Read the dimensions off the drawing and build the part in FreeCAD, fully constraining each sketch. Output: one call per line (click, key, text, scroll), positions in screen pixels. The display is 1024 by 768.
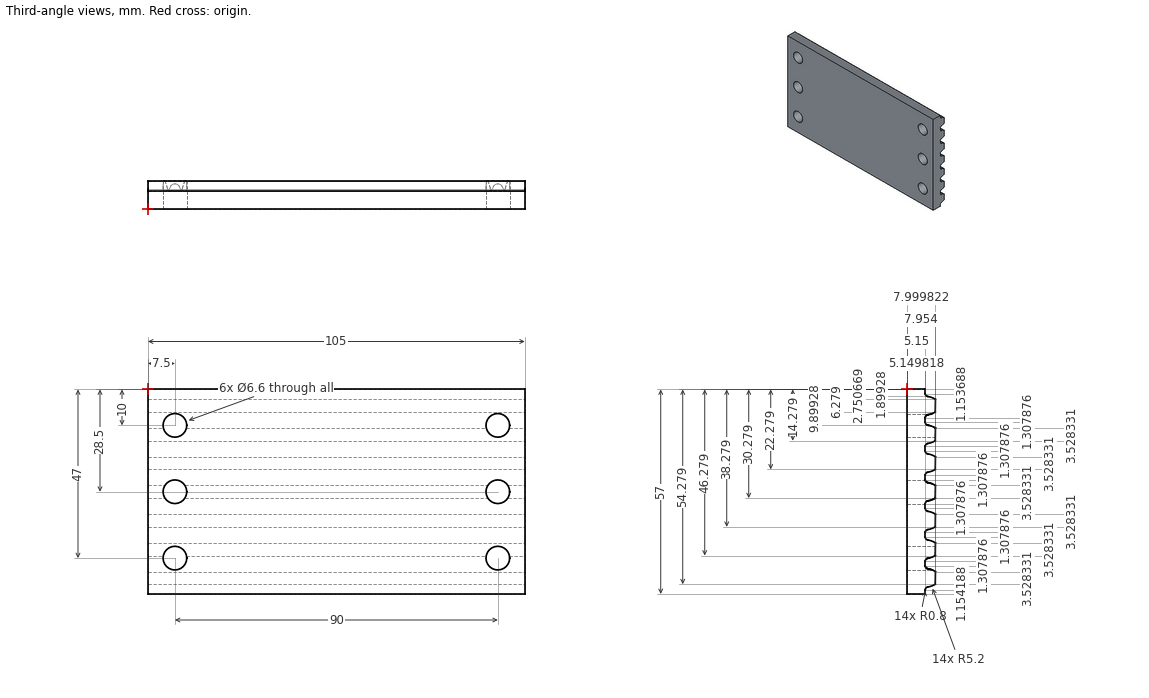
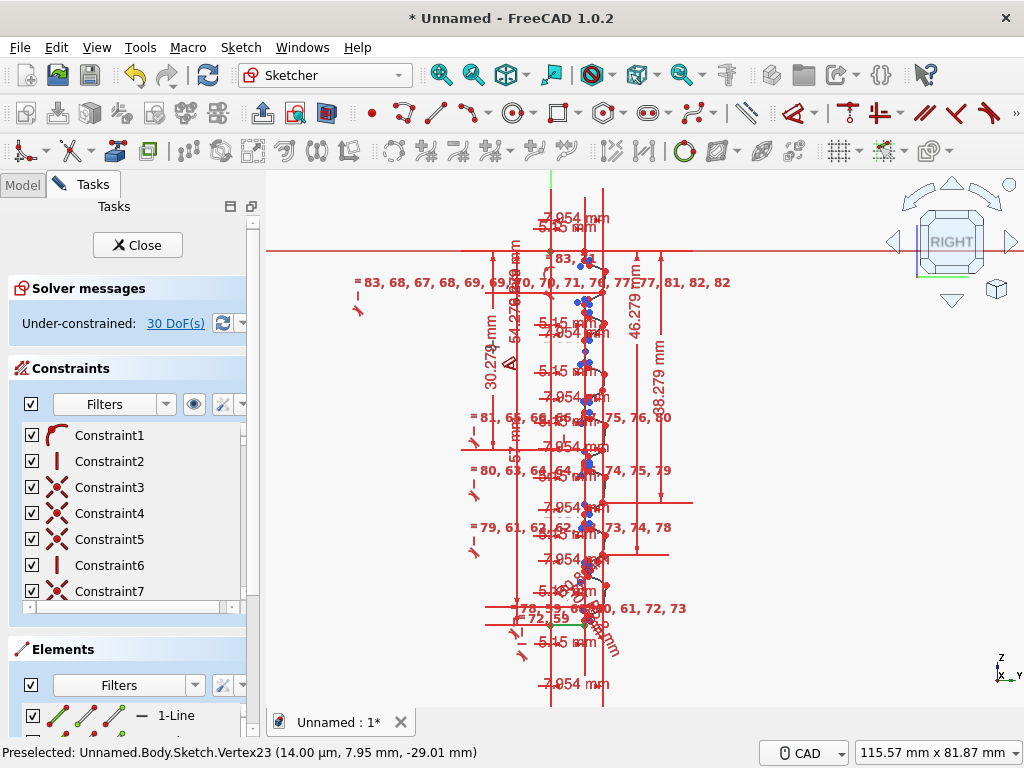
click(603, 390)
click(637, 272)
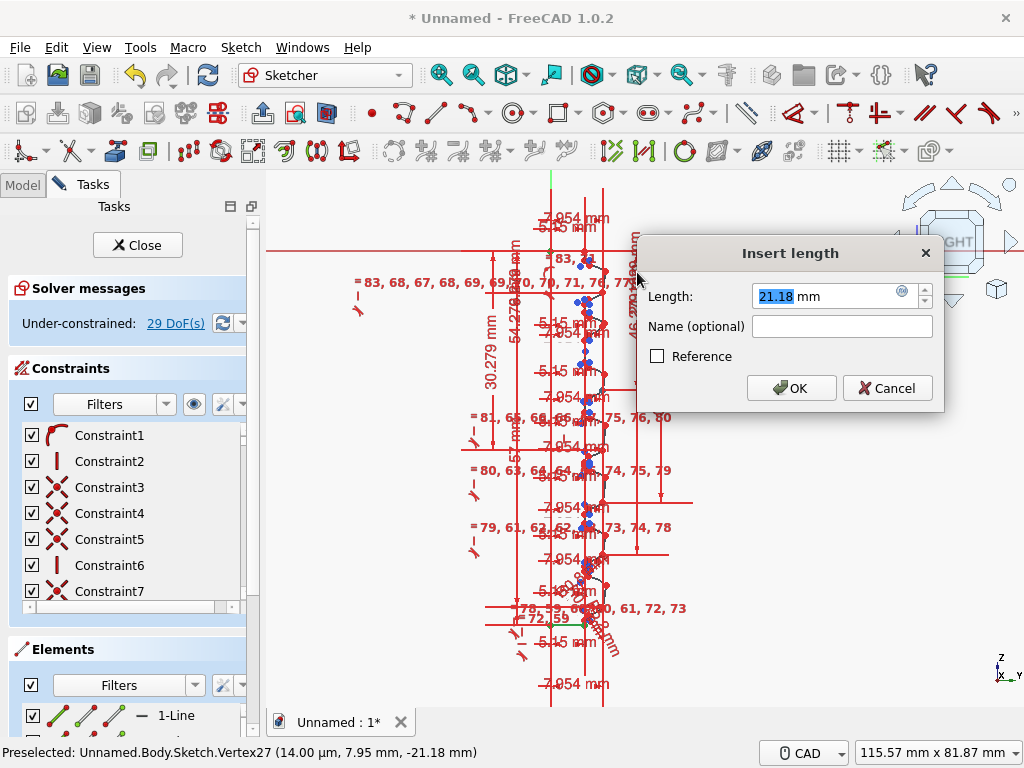
text(22.279)
key(Return)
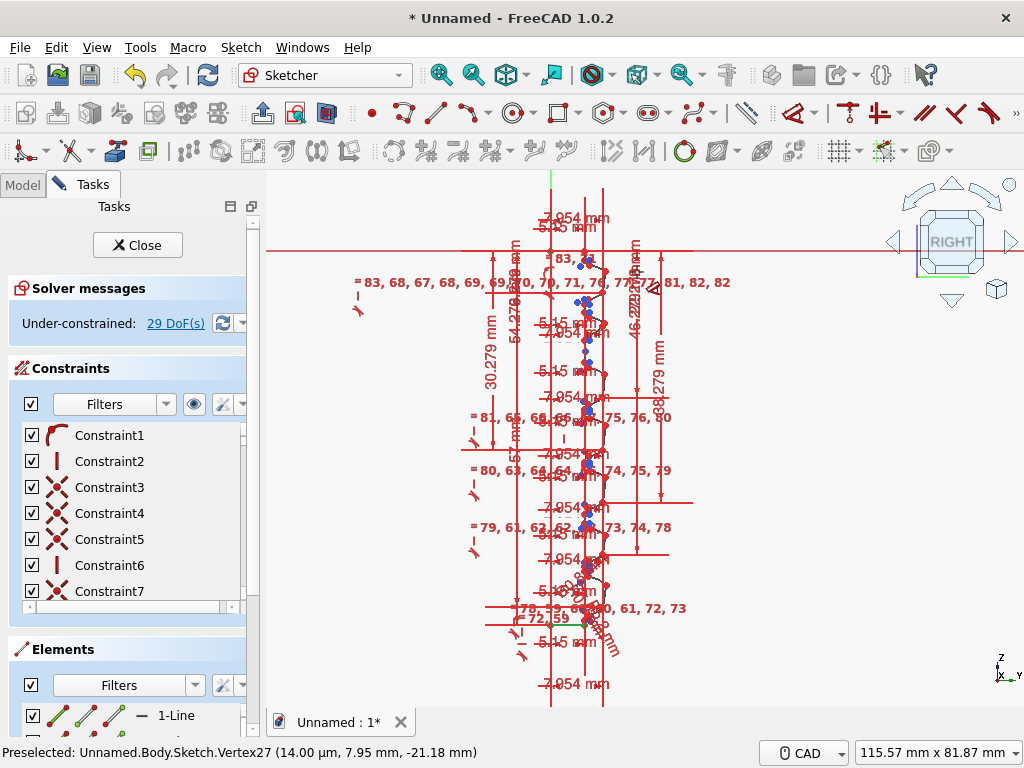
scroll(603, 326, up, 7)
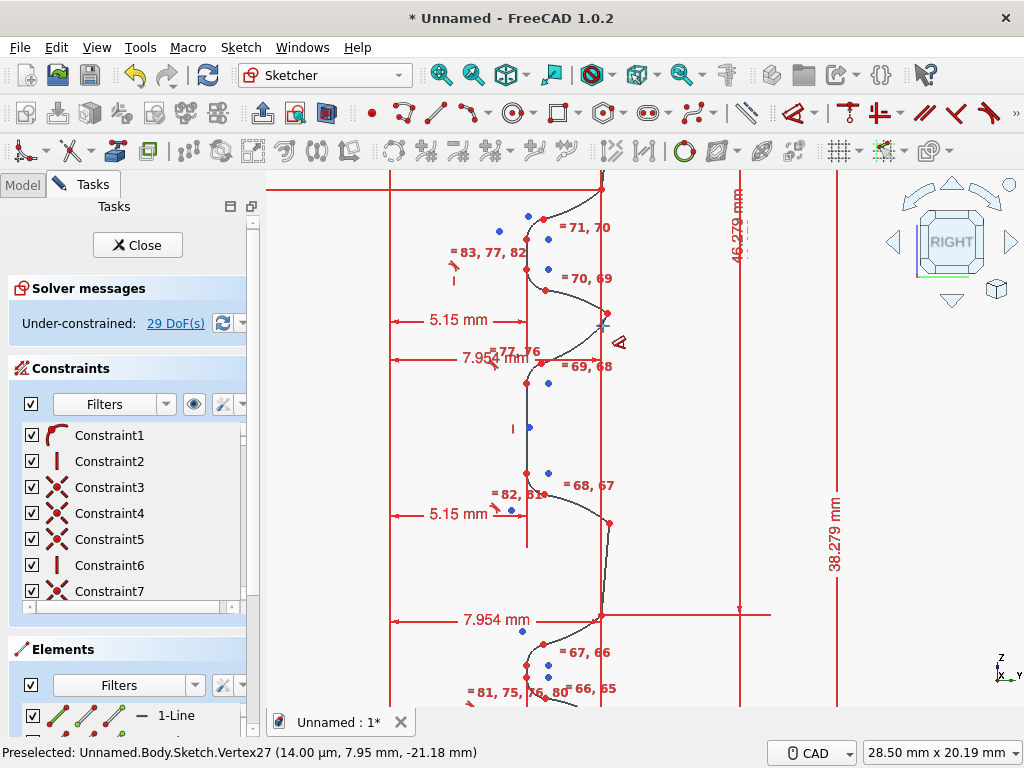
click(601, 325)
click(356, 262)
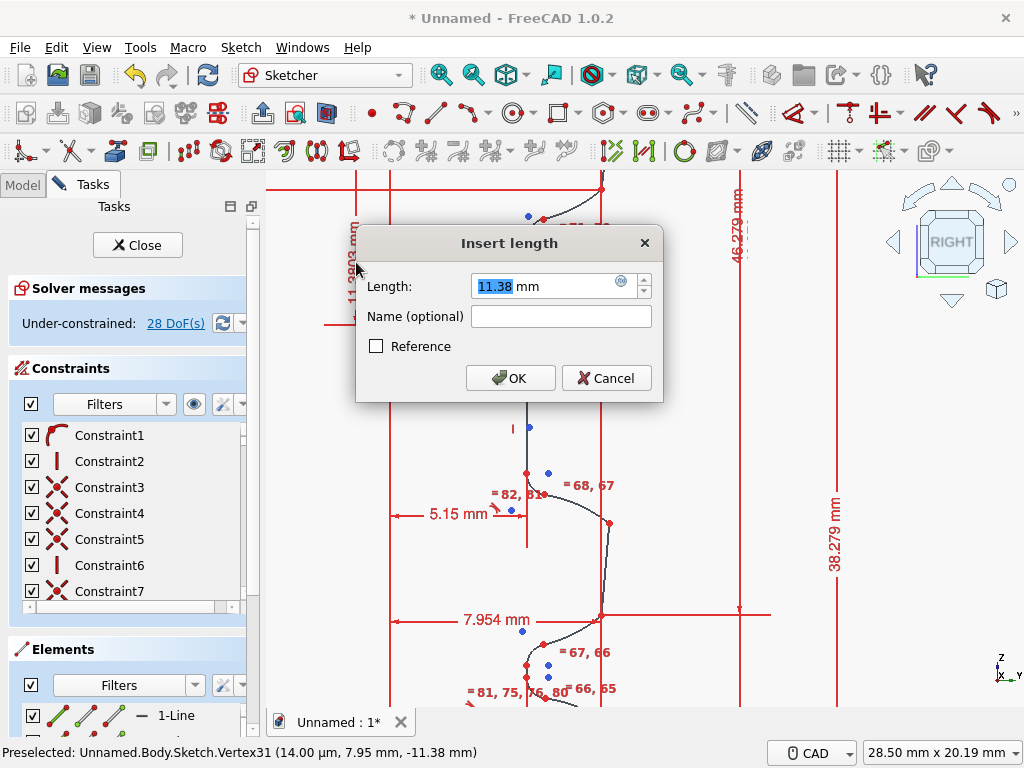
text(14.279)
key(Return)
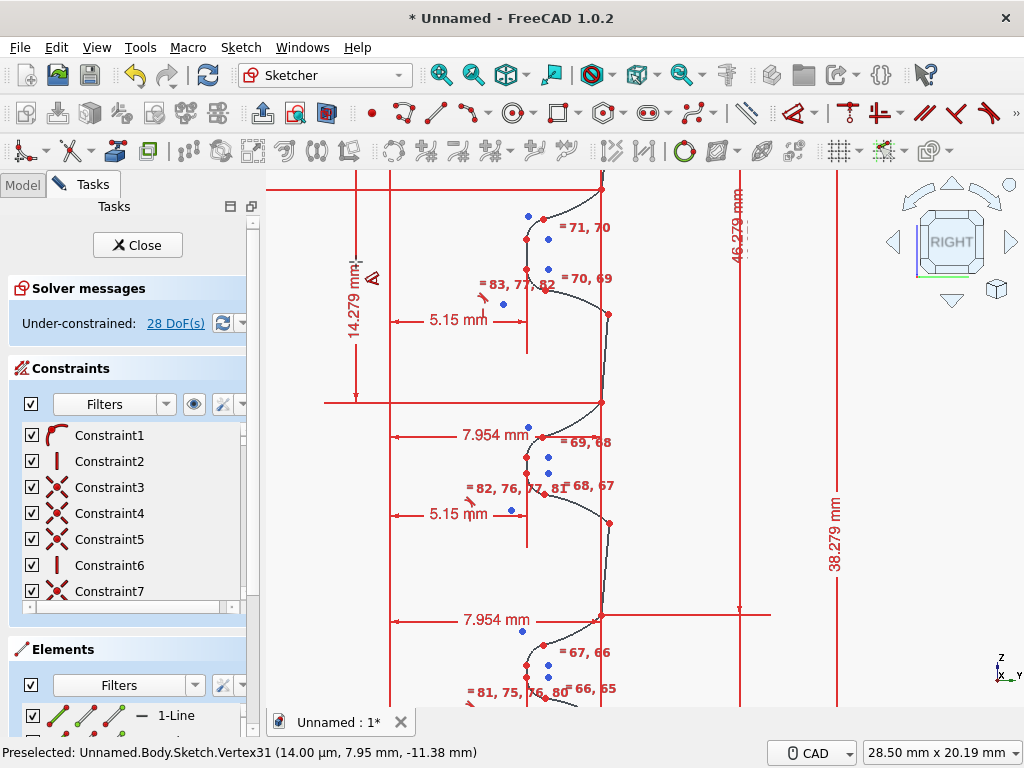
scroll(603, 326, down, 7)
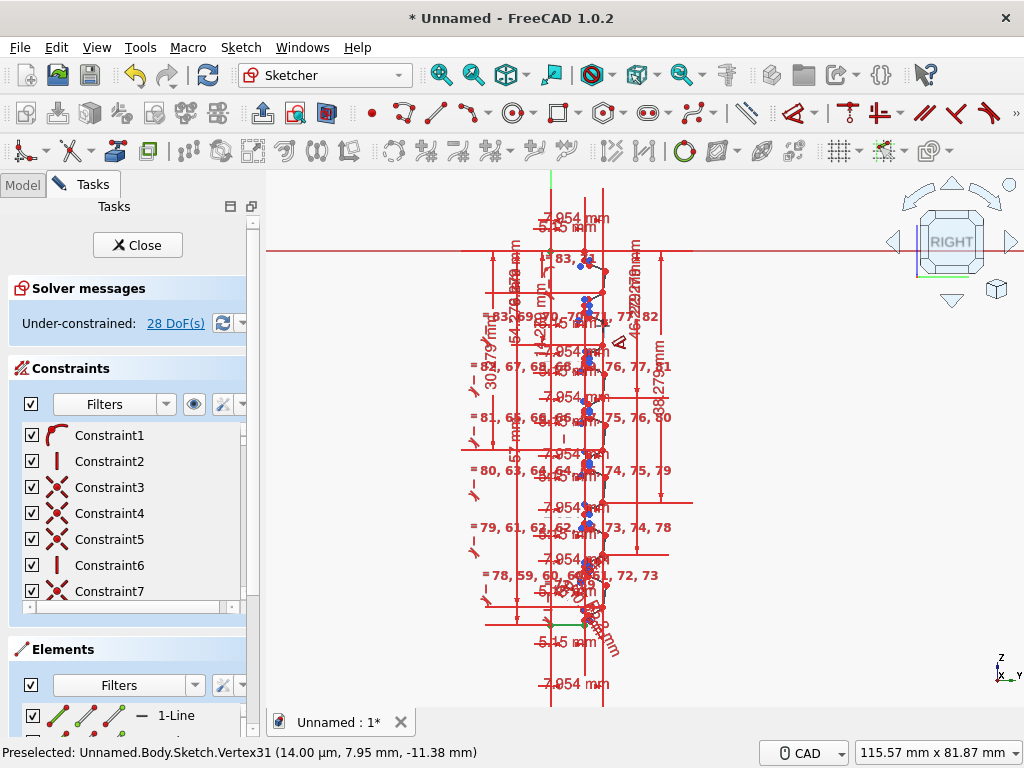
scroll(585, 257, up, 9)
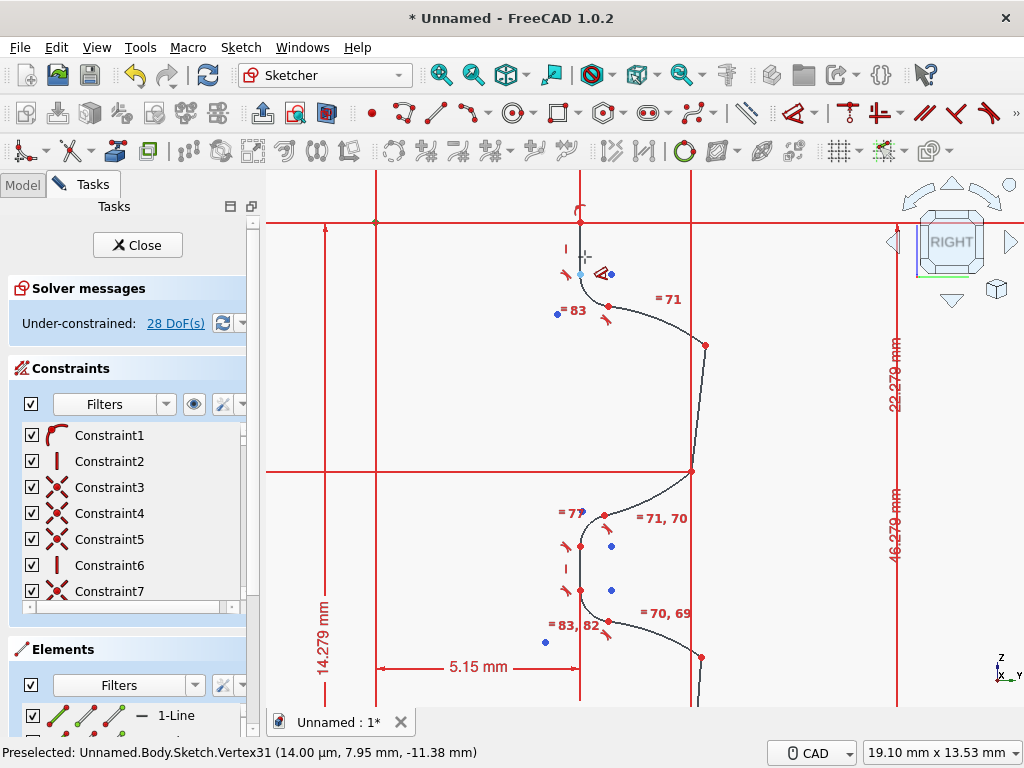
click(580, 259)
click(614, 249)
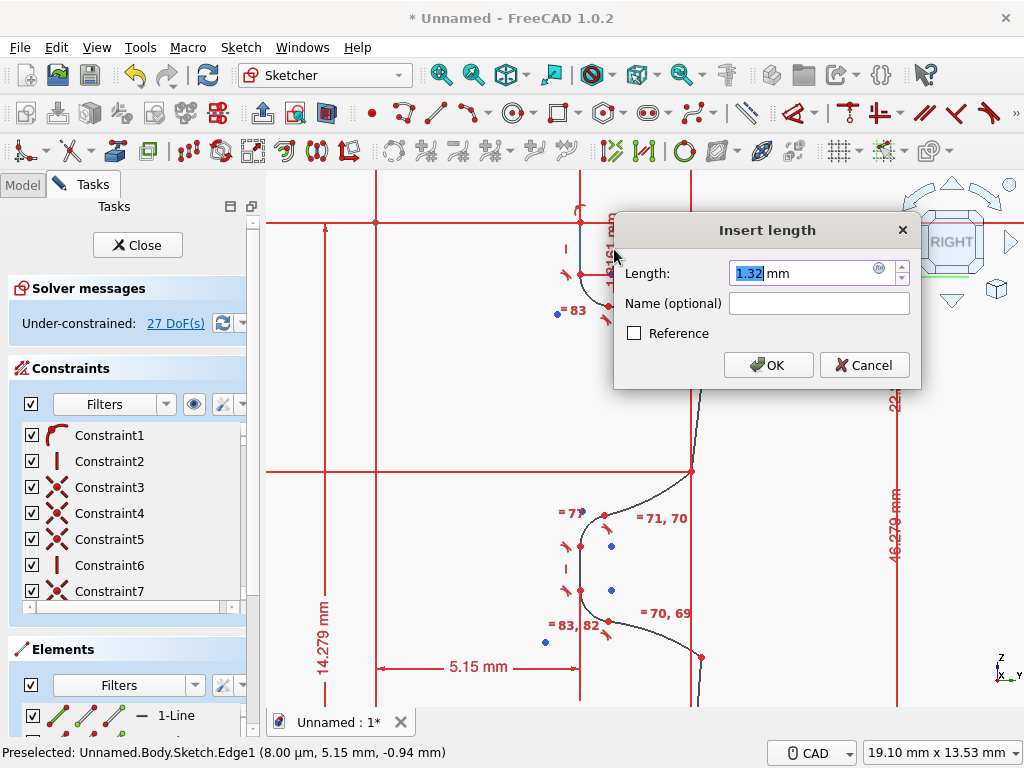
text(1.153688)
key(Return)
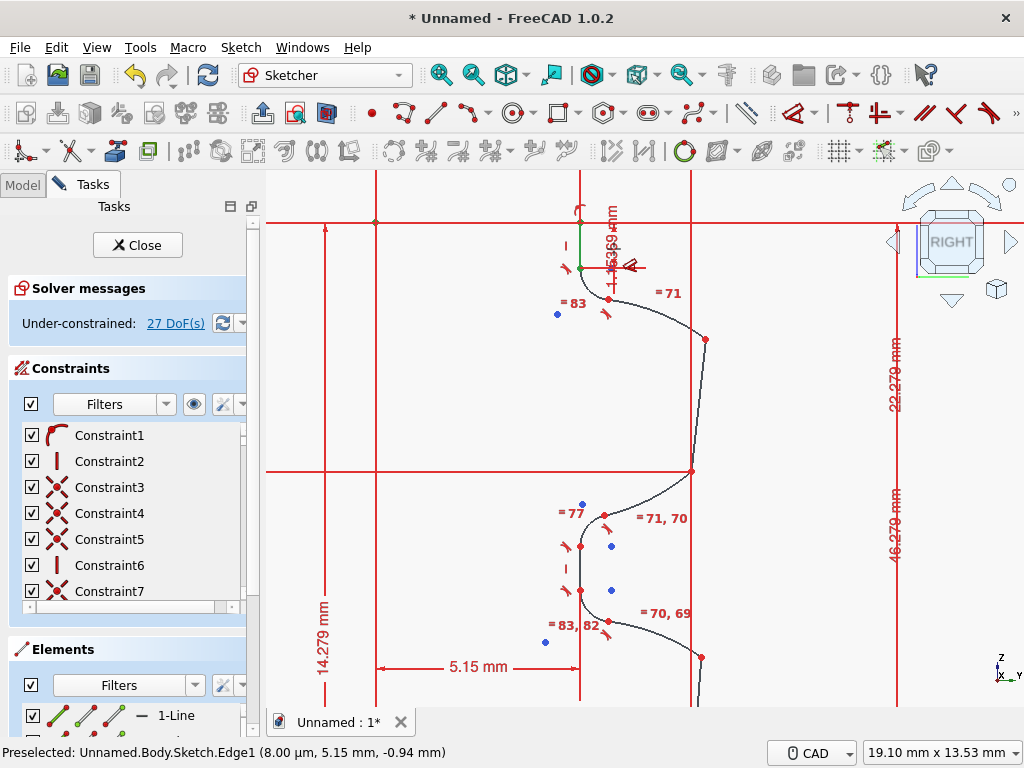
scroll(585, 257, down, 9)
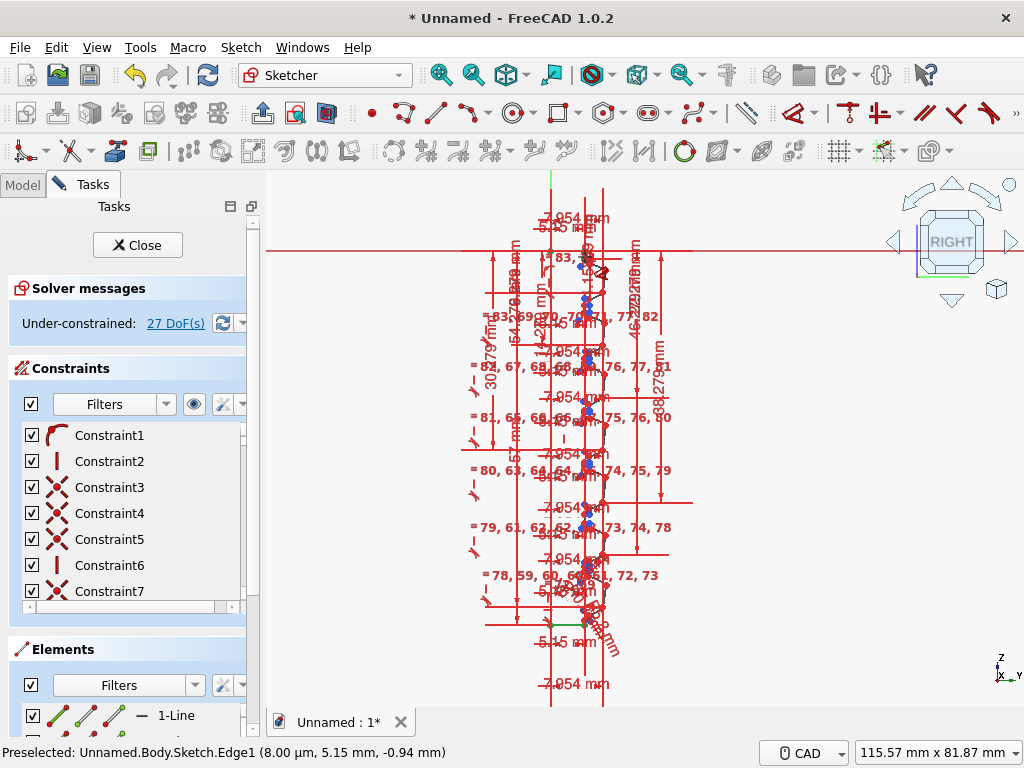
scroll(585, 624, up, 12)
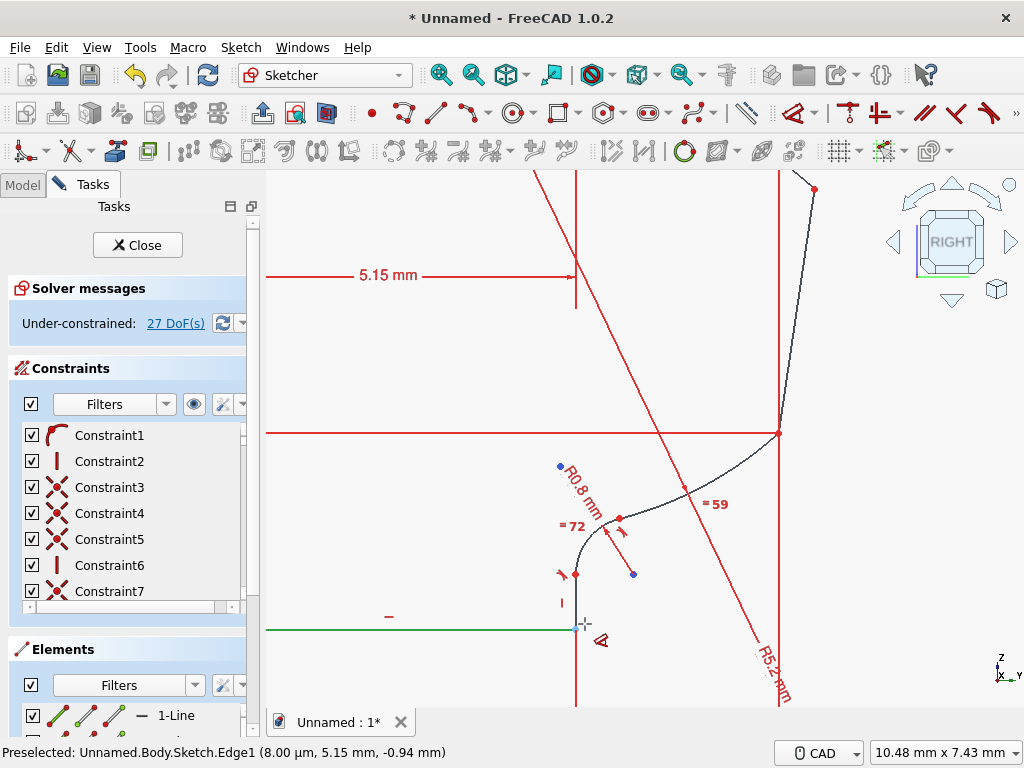
click(576, 613)
click(610, 602)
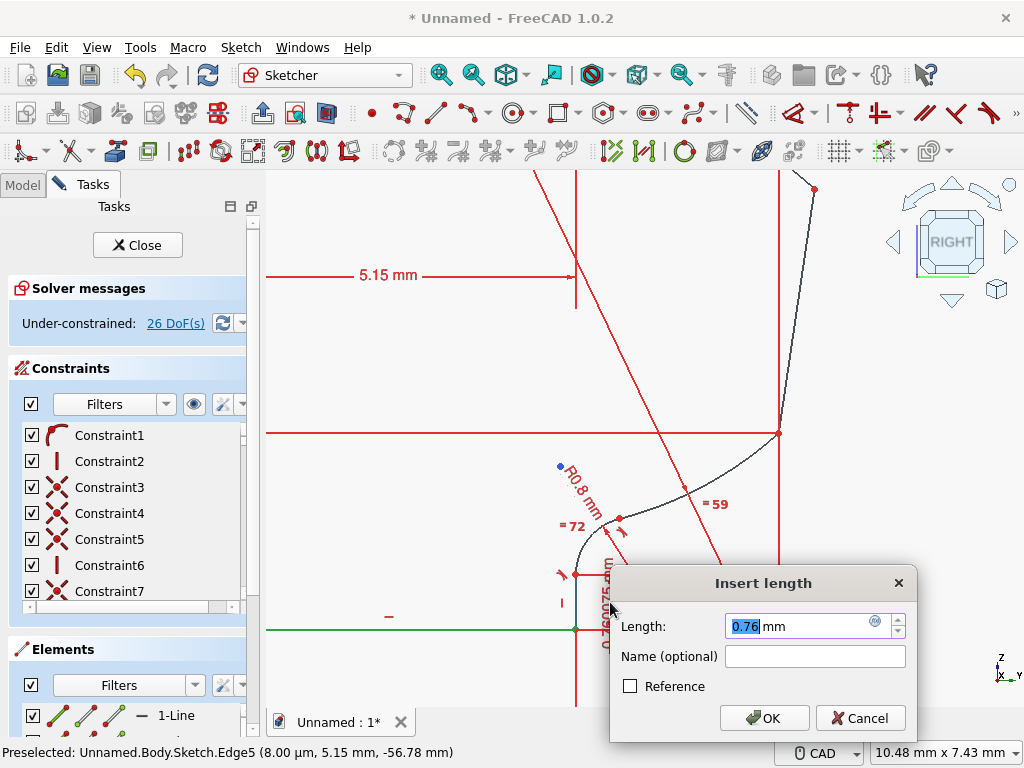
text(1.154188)
key(Return)